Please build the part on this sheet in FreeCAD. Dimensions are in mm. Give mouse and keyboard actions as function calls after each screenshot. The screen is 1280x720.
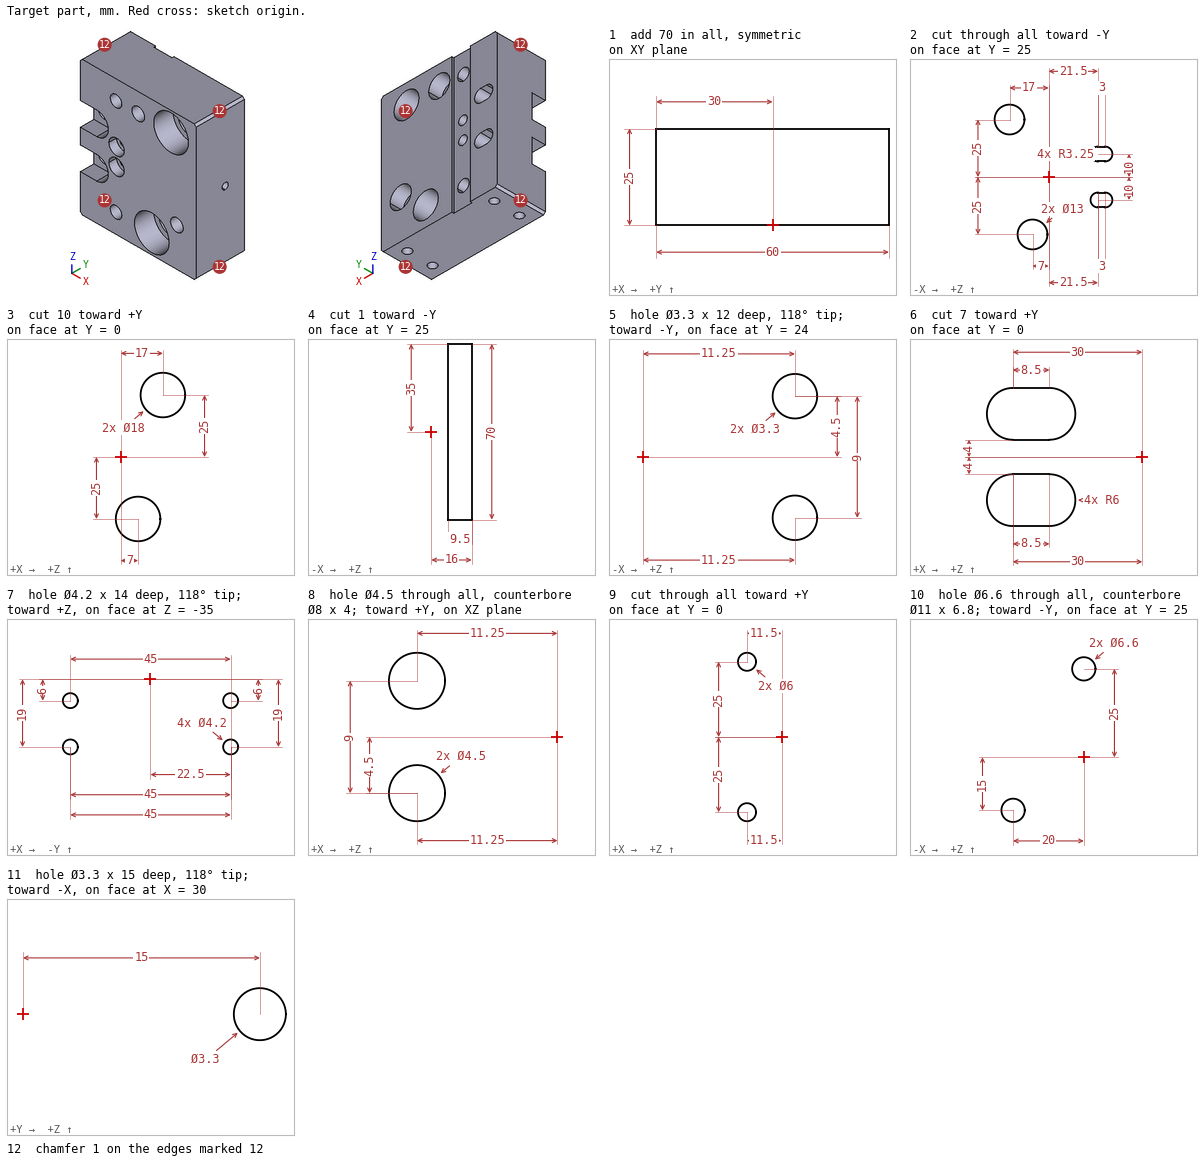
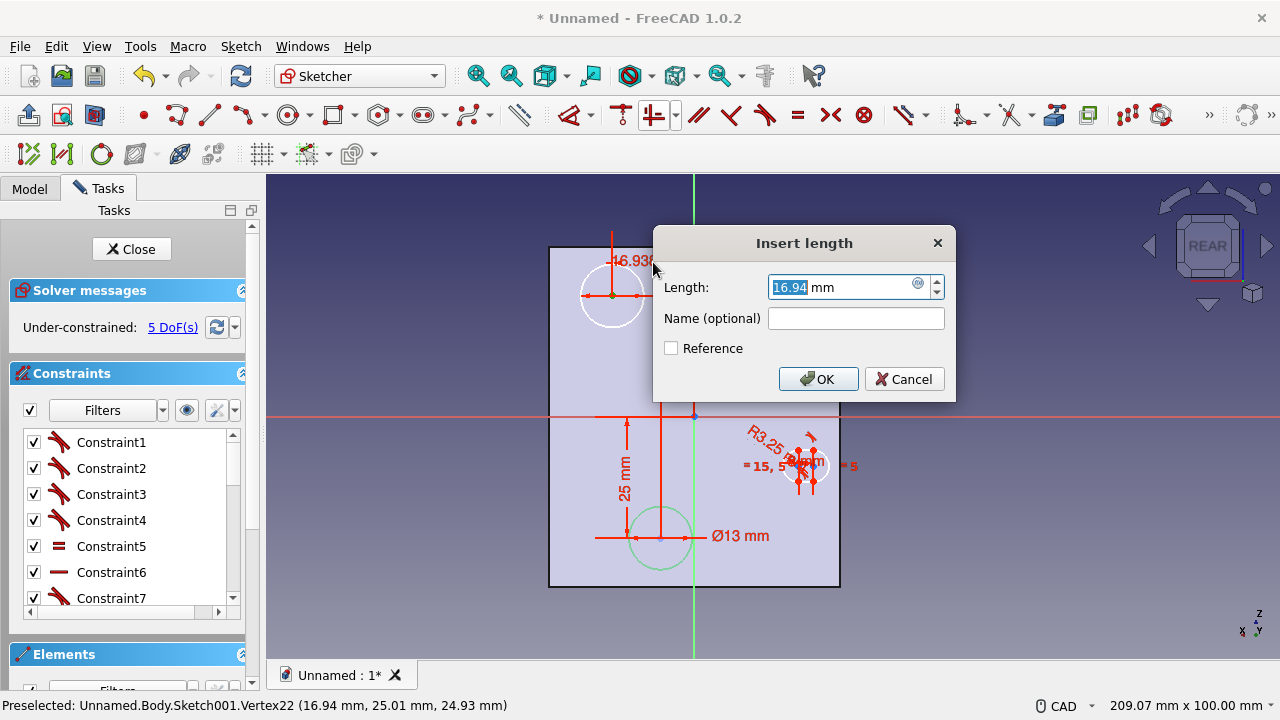
text(17)
key(Return)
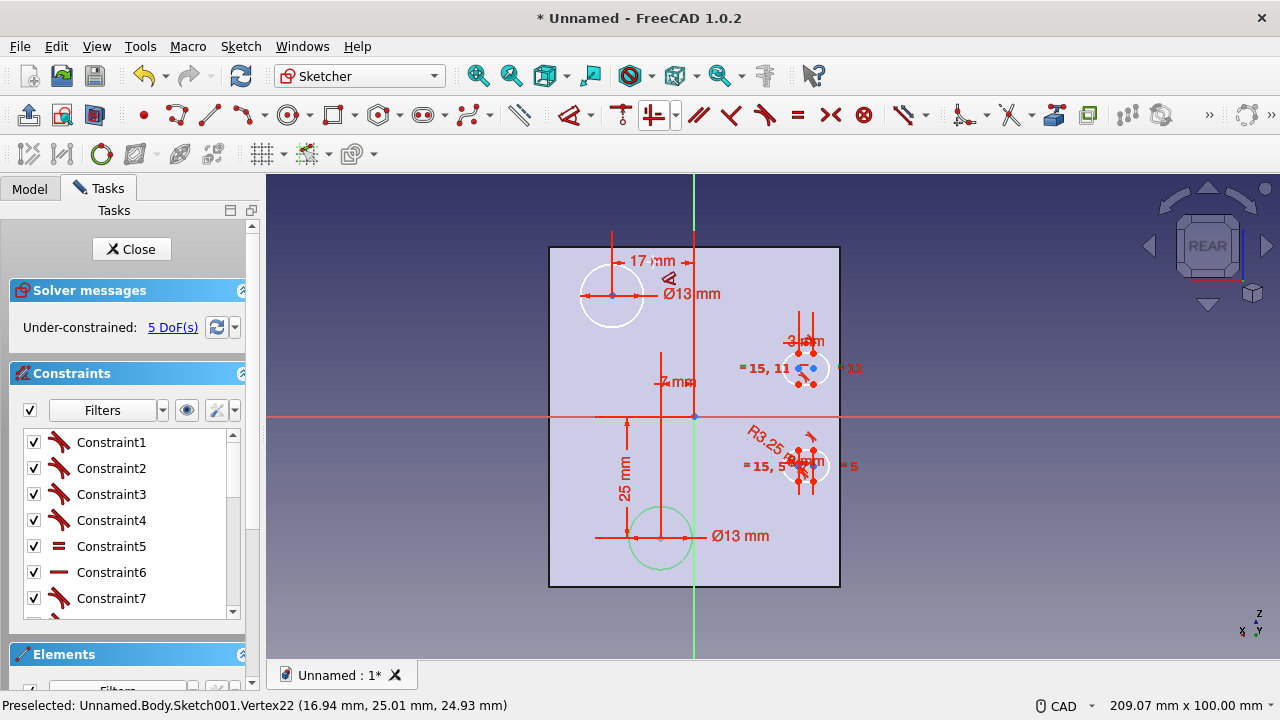
click(612, 296)
click(578, 356)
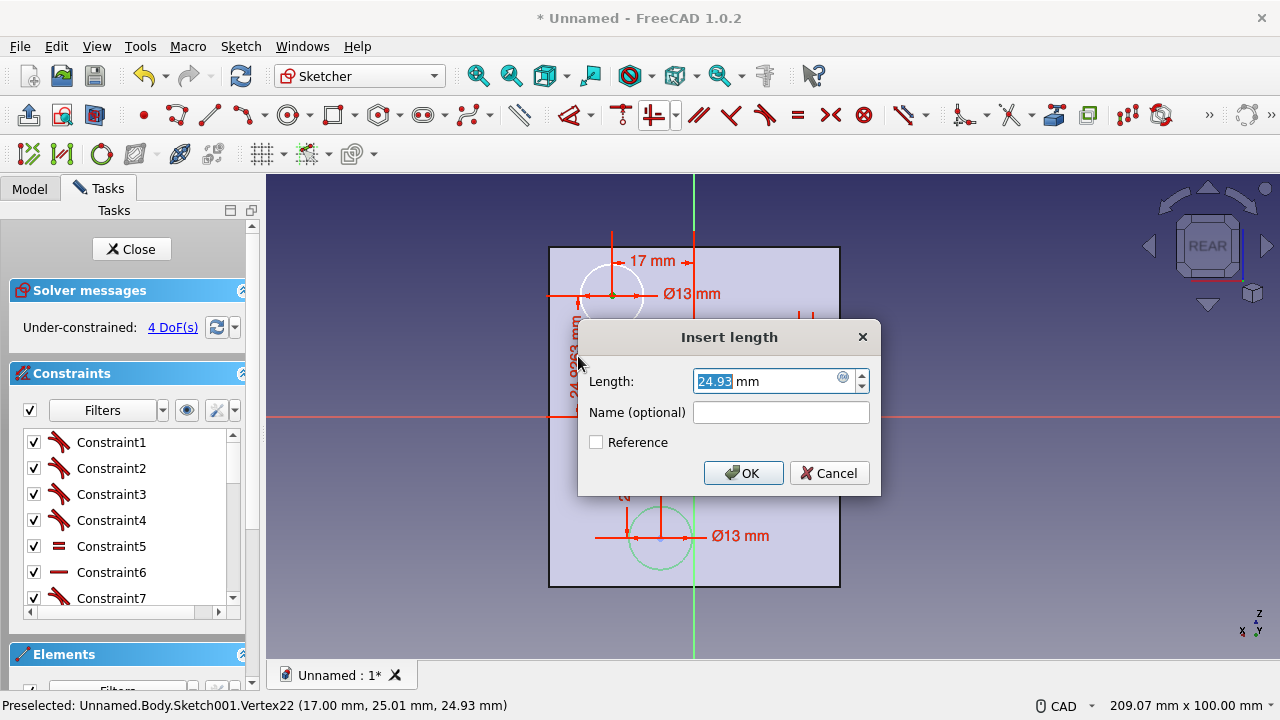
text(25)
key(Return)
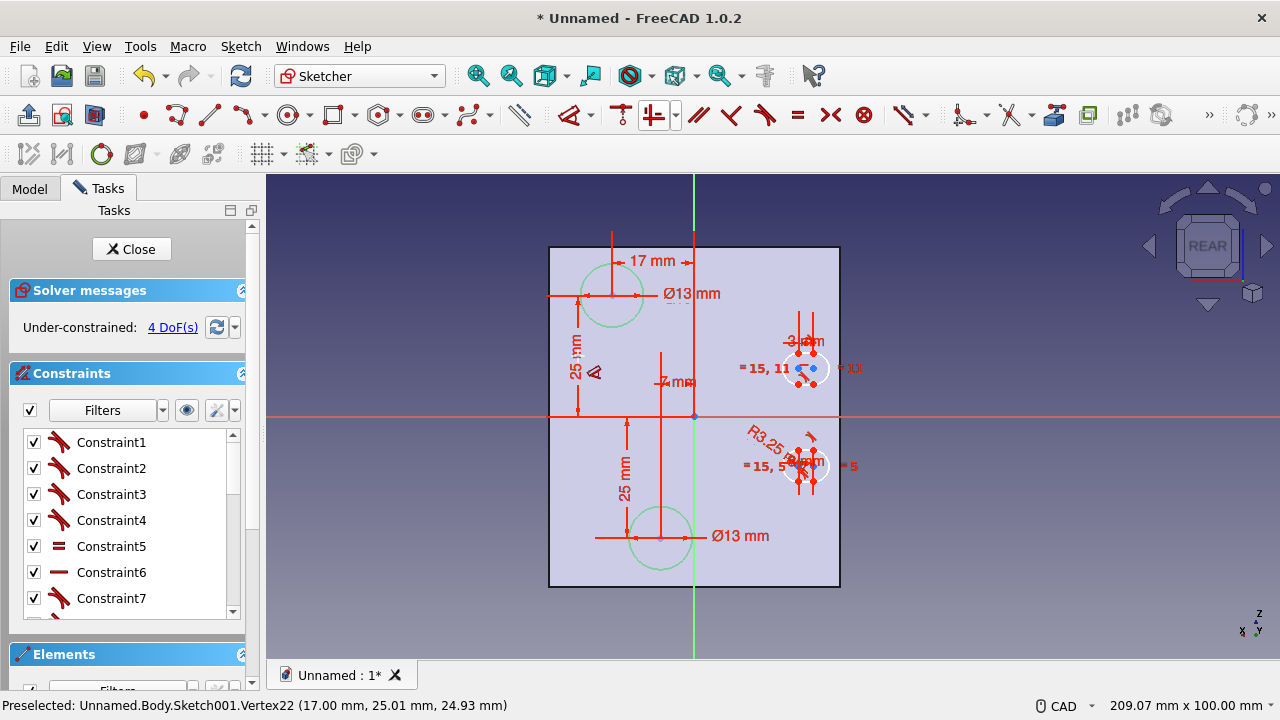
click(799, 466)
click(660, 442)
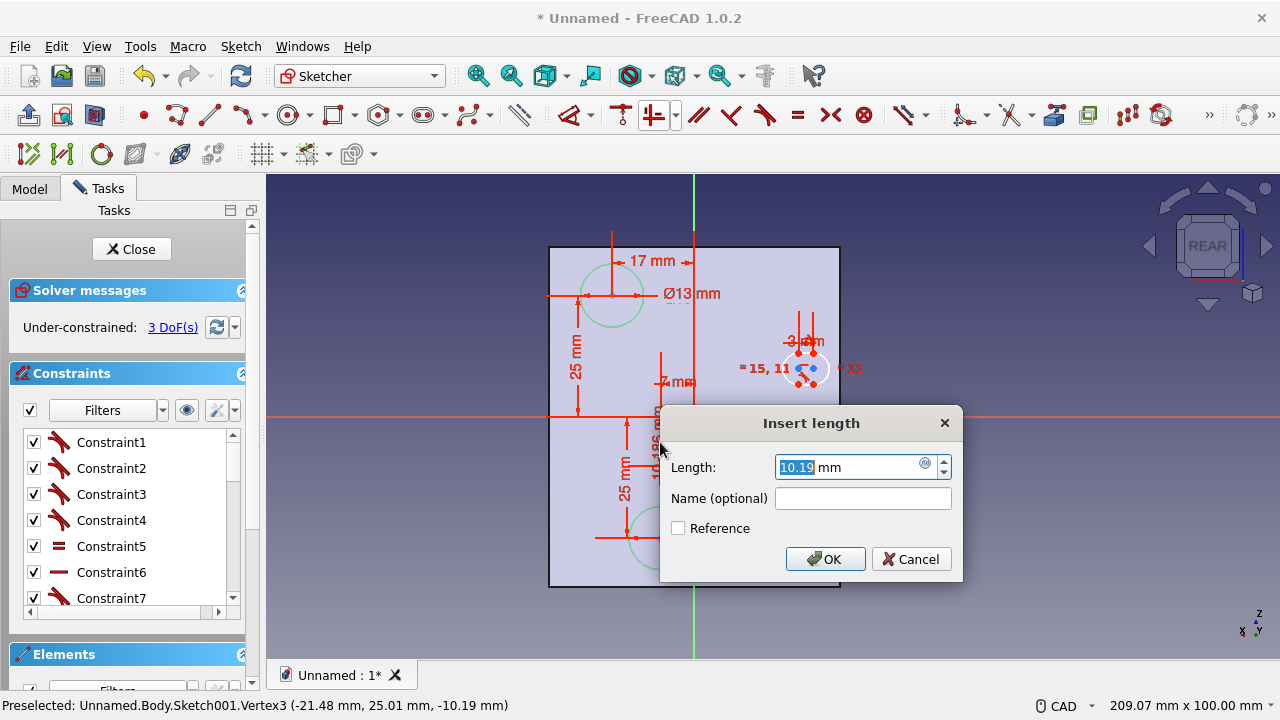
text(10)
key(Return)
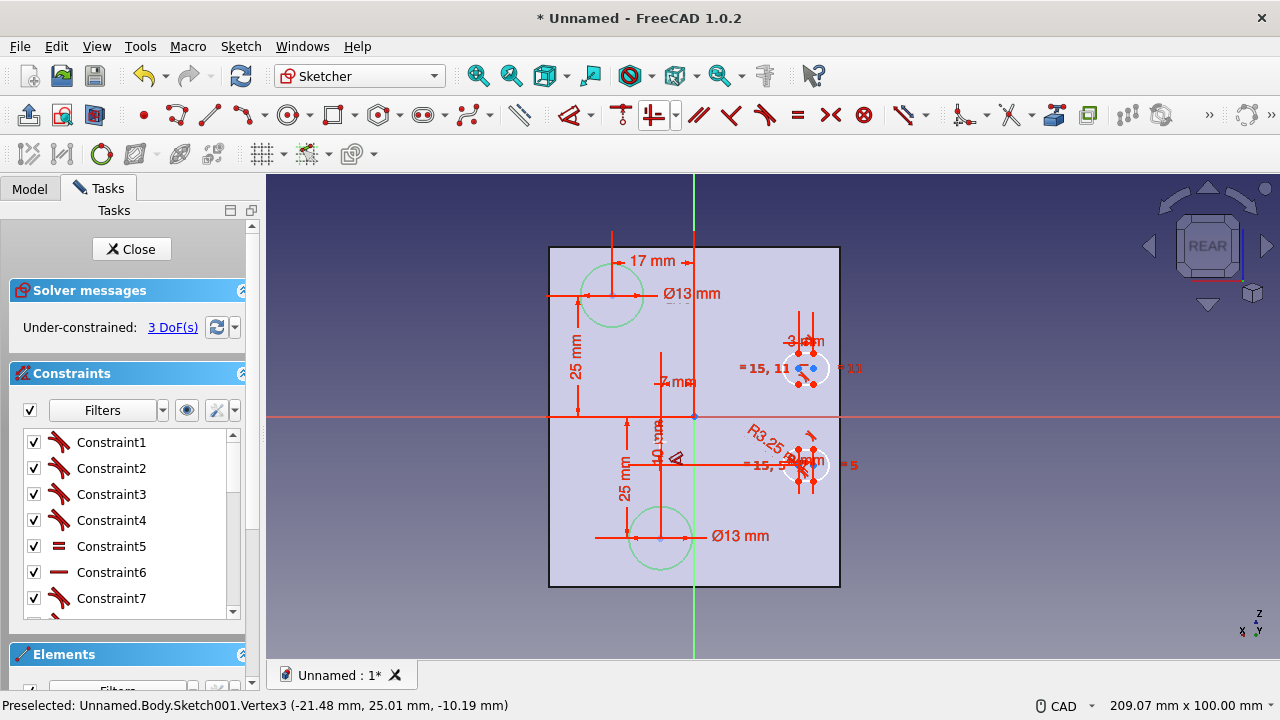
click(799, 369)
click(833, 393)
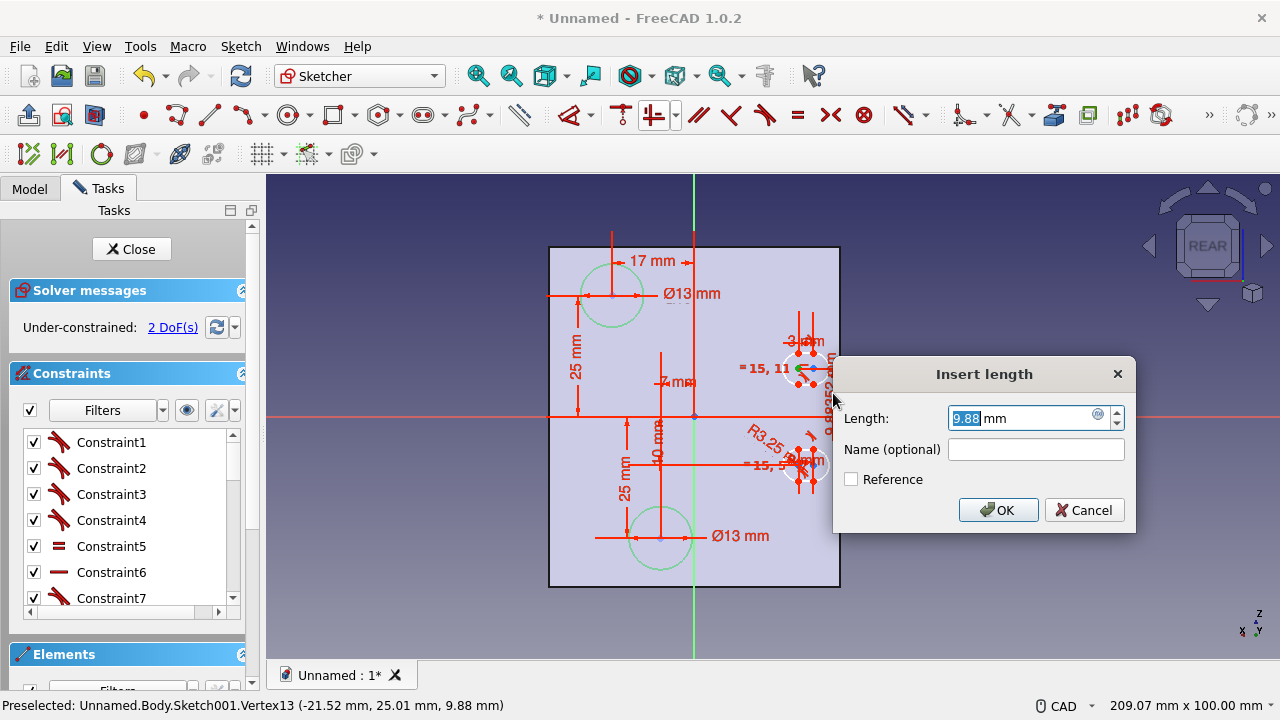
text(10)
key(Return)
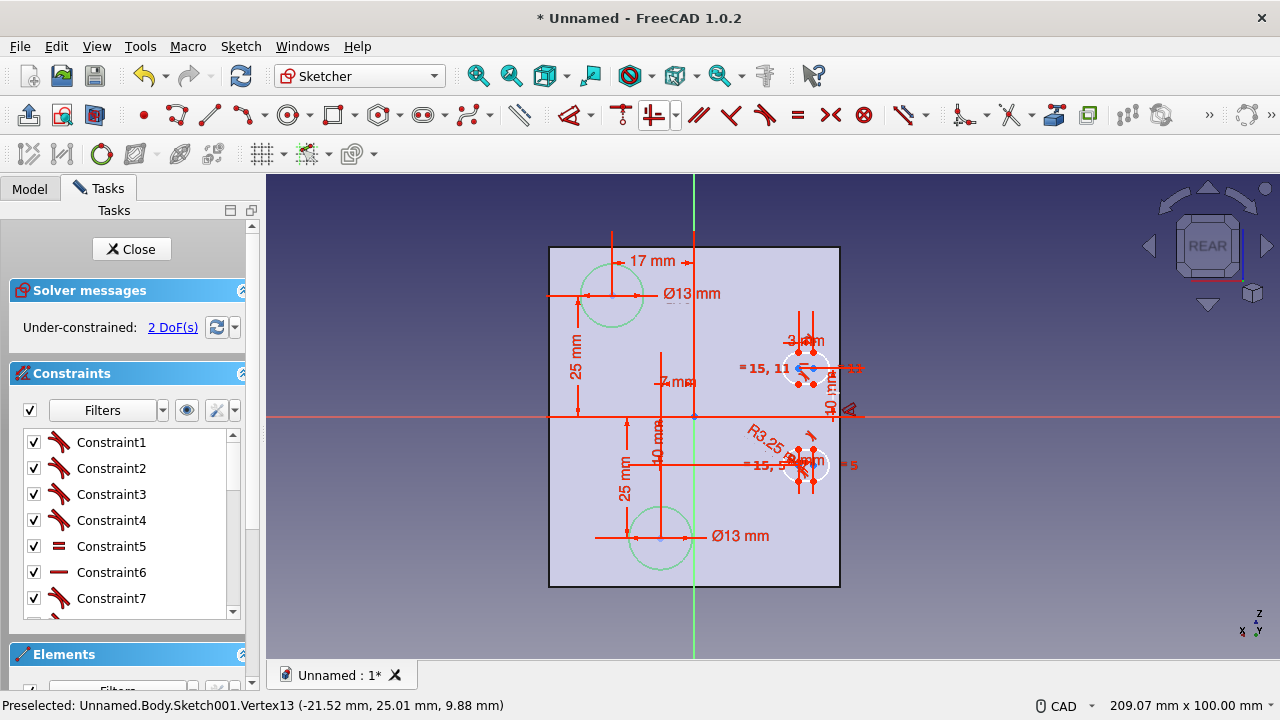
click(799, 450)
click(747, 484)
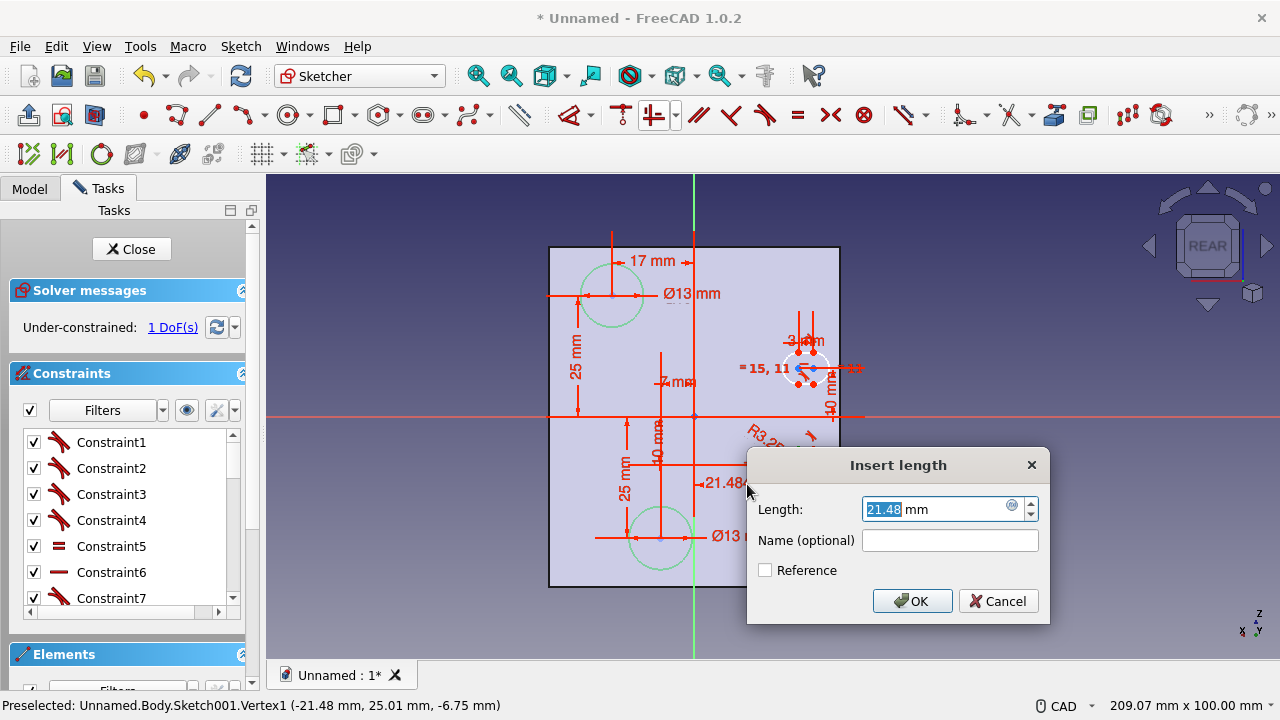
text(21.5)
key(Return)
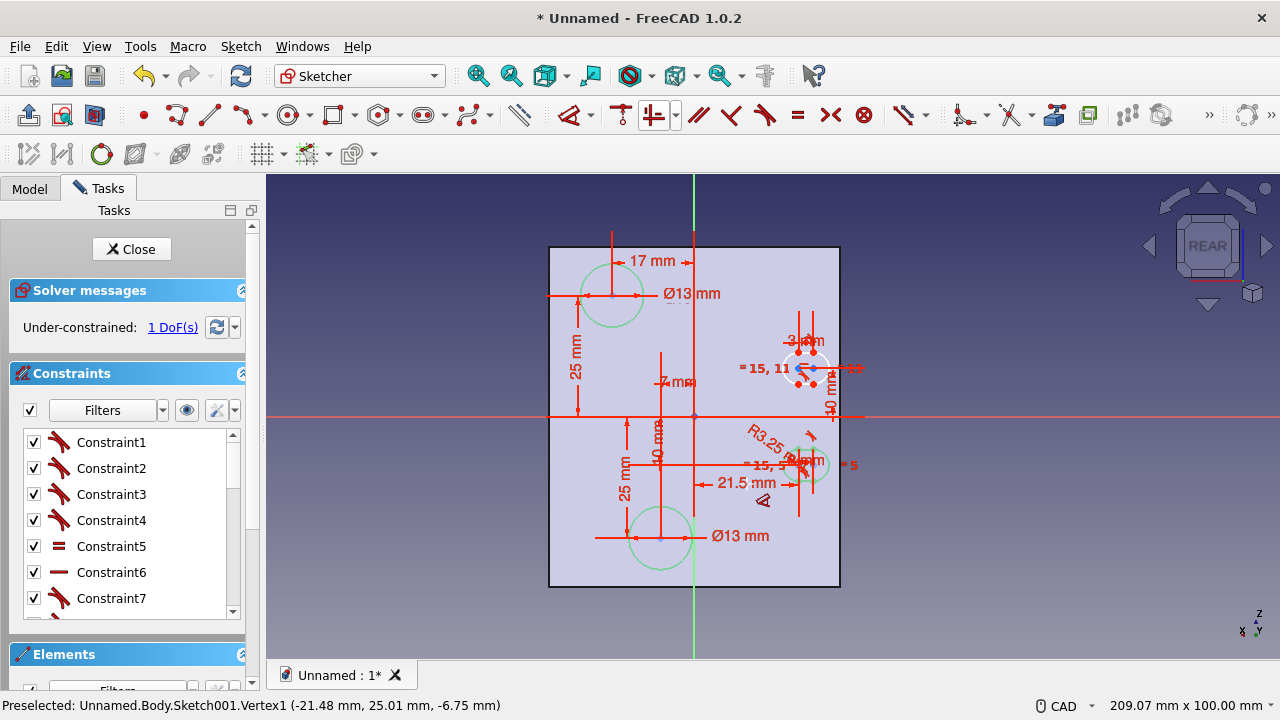
click(799, 353)
click(747, 319)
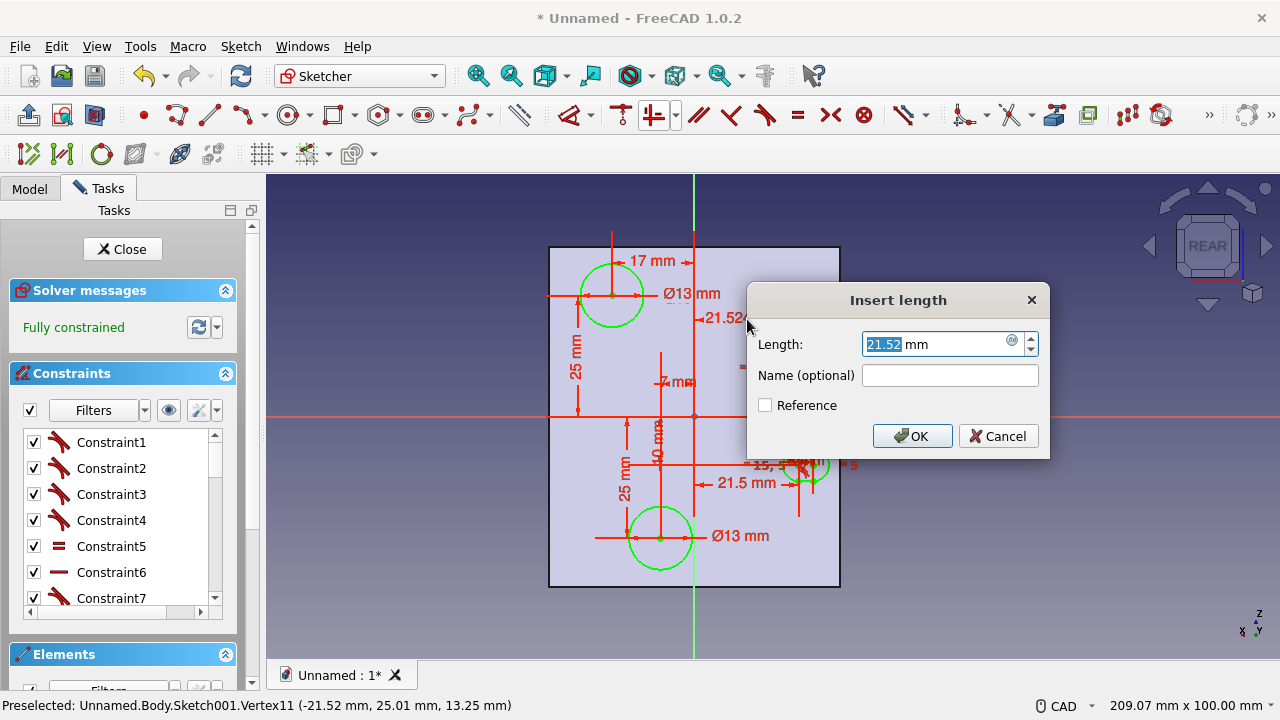
text(21.5)
key(Return)
key(Escape)